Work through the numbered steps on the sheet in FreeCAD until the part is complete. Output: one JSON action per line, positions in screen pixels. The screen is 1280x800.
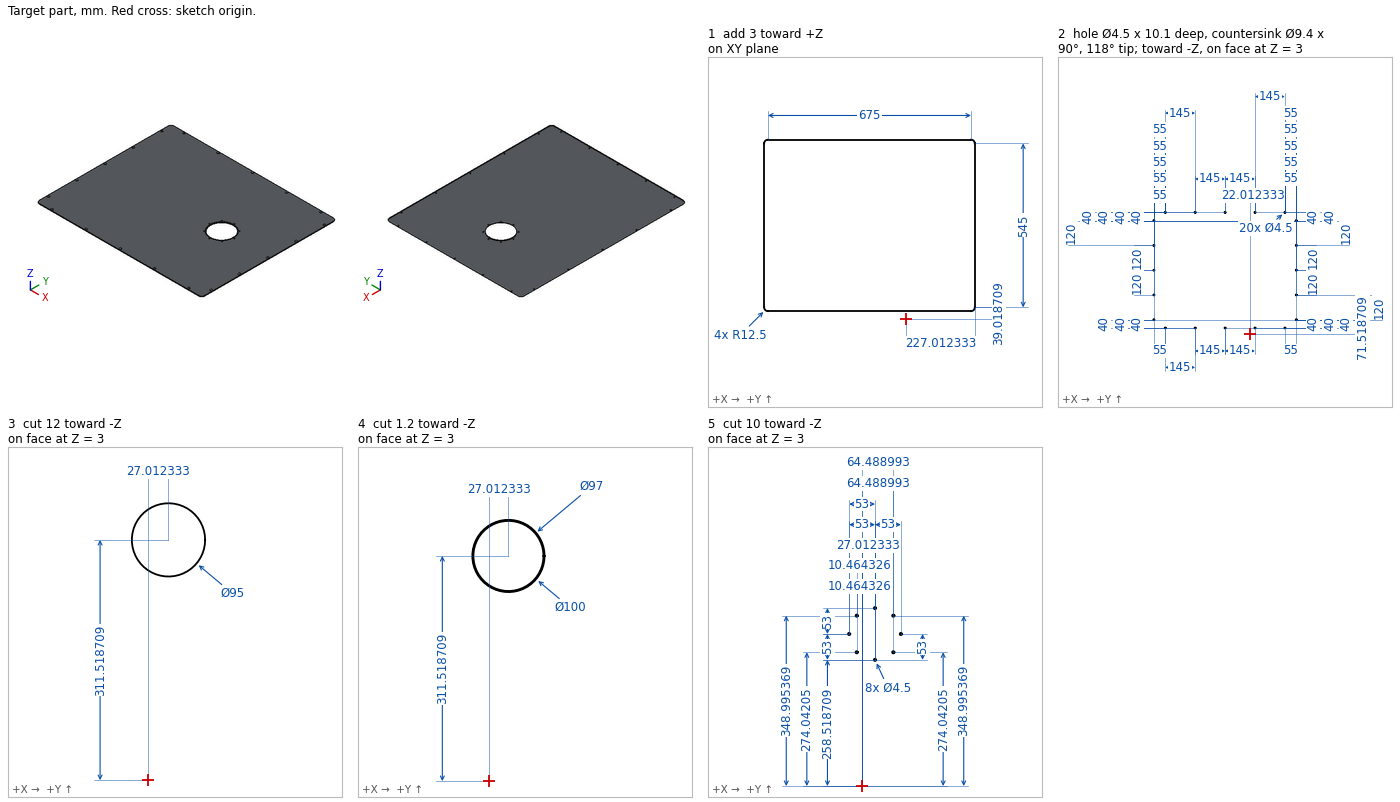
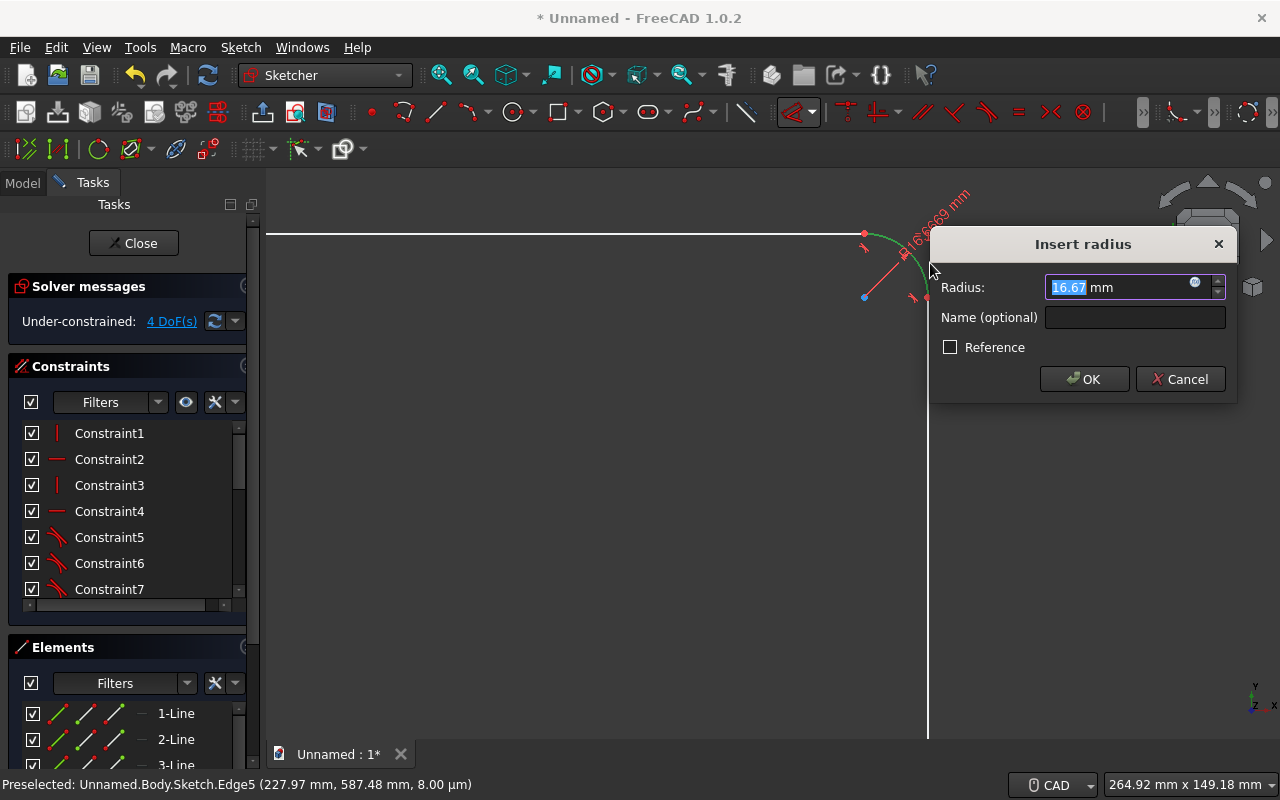
{"action": "type", "text": "12.5"}
{"action": "key", "text": "Return"}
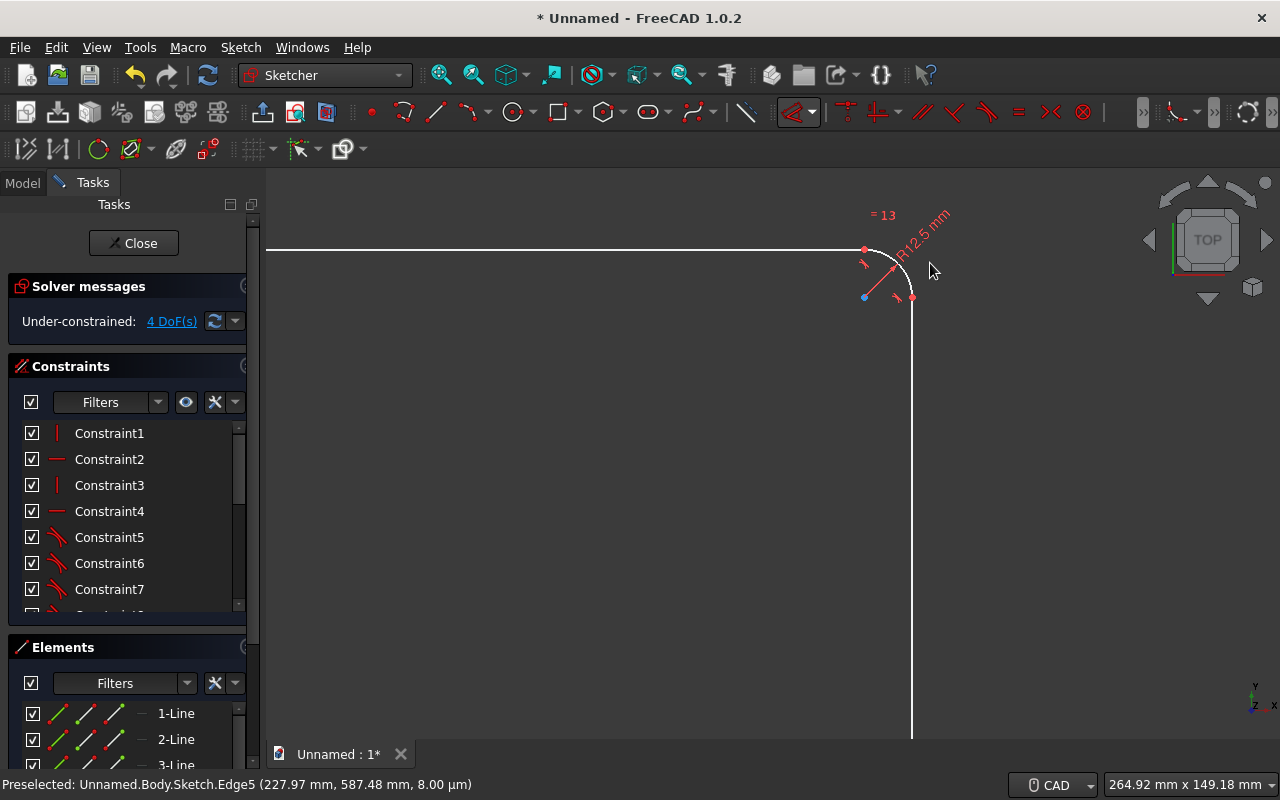
{"action": "scroll", "coordinate": [927, 270], "scroll_direction": "down", "scroll_amount": 9}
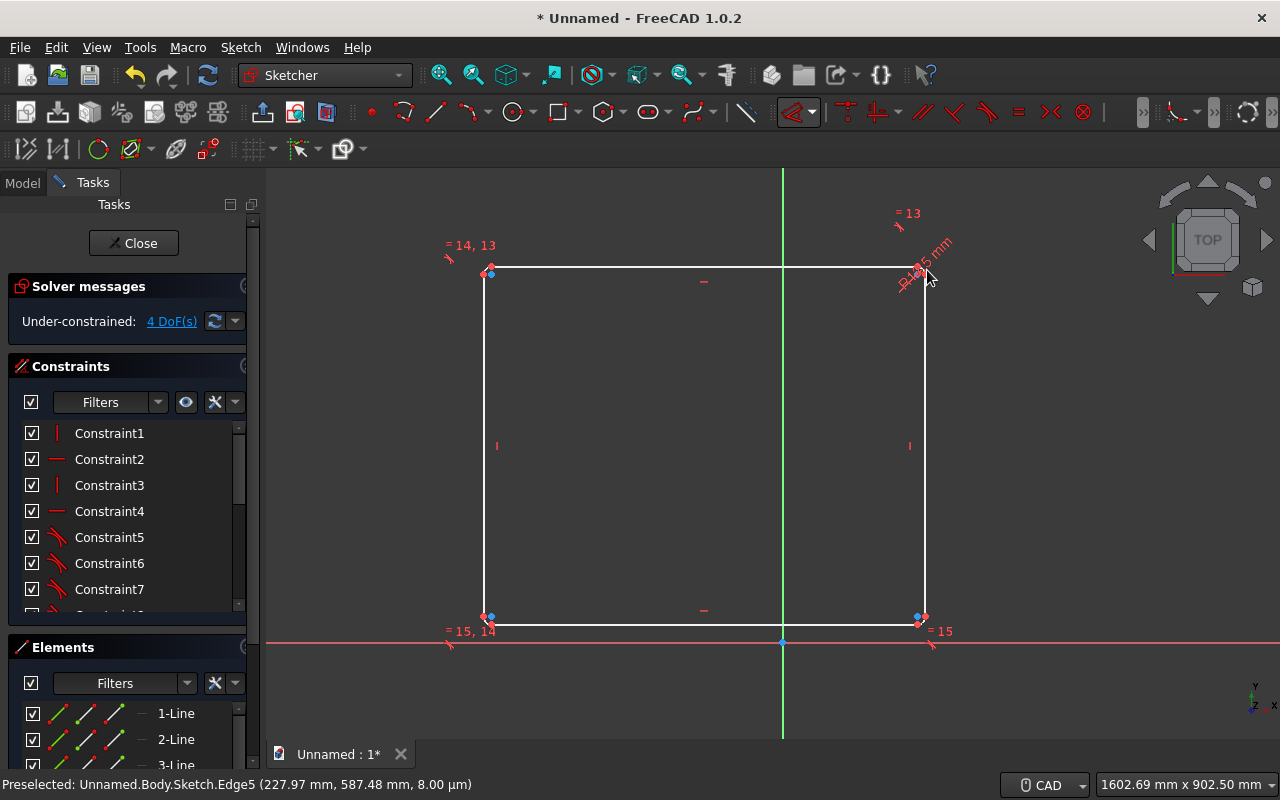
{"action": "left_click", "coordinate": [925, 514]}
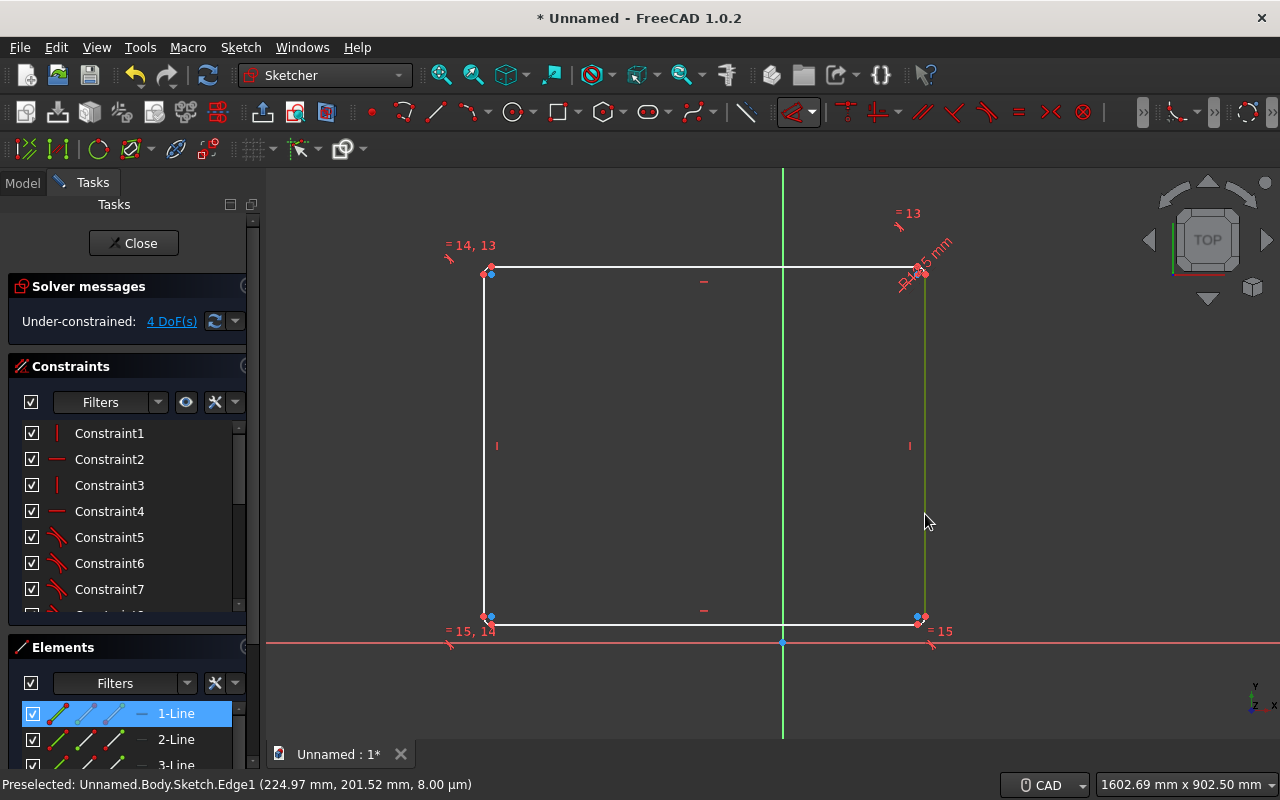
{"action": "key", "text": "i"}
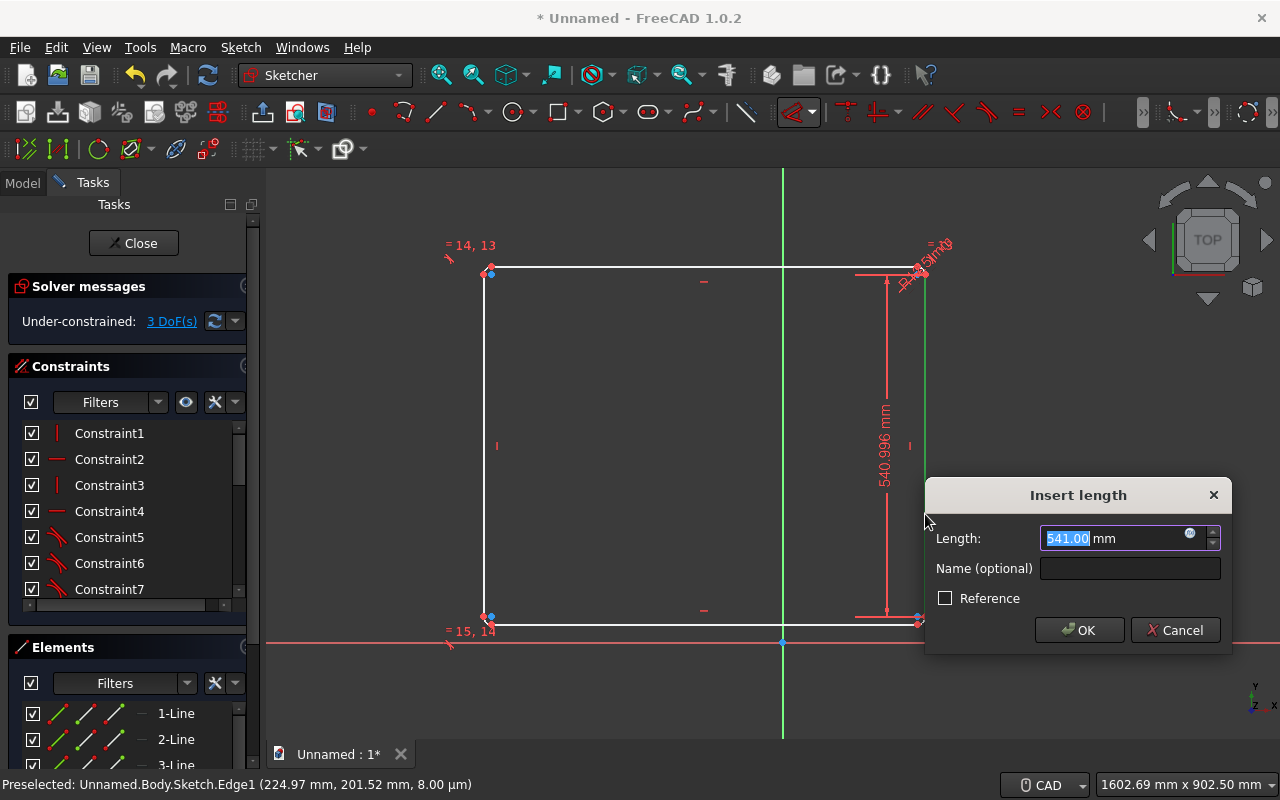
{"action": "type", "text": "545"}
{"action": "key", "text": "Return"}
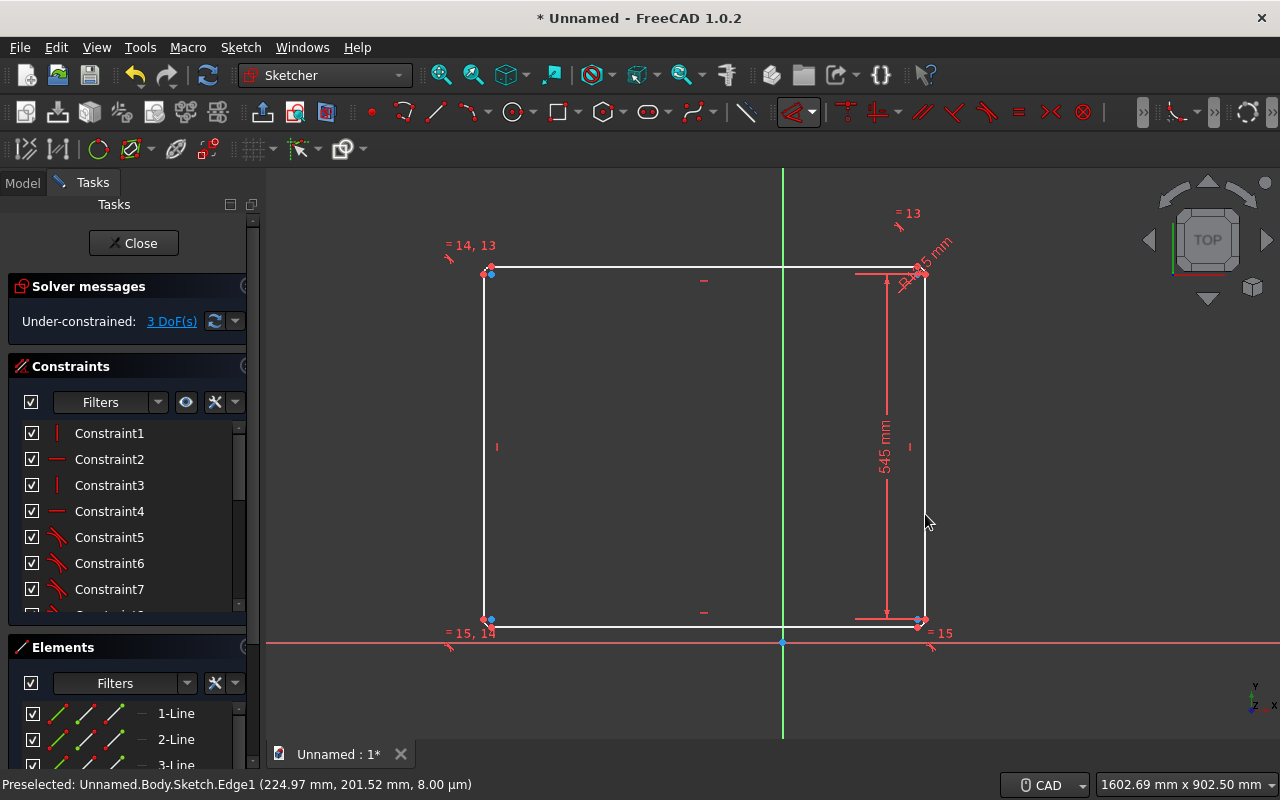
{"action": "left_click", "coordinate": [619, 267]}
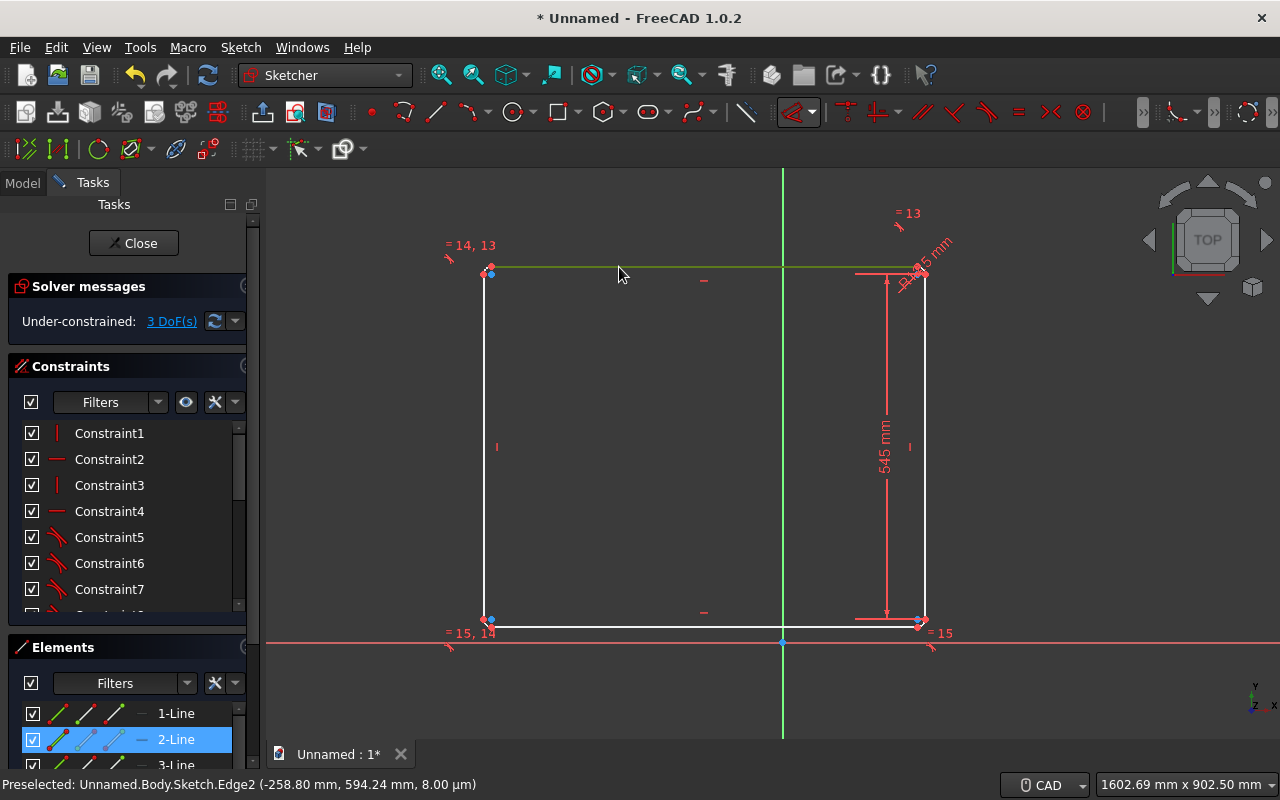
{"action": "left_click", "coordinate": [814, 112]}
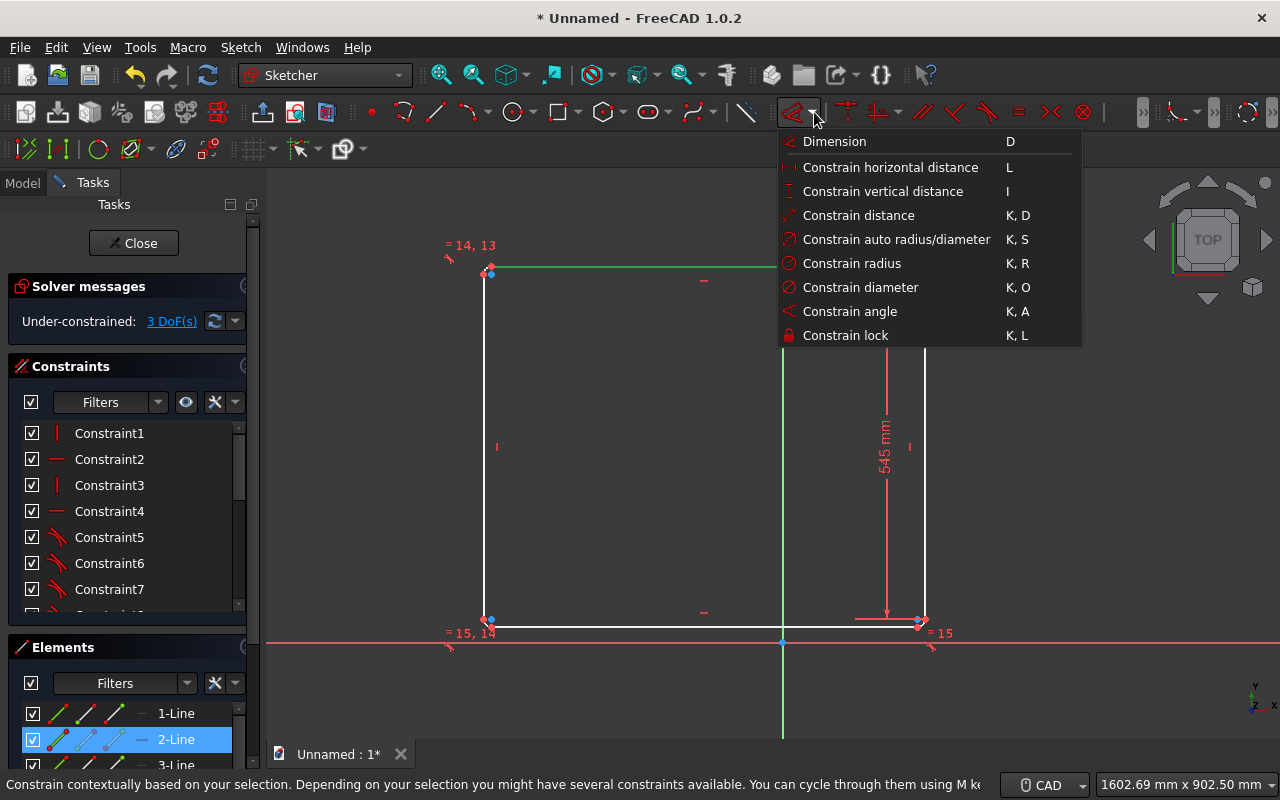
{"action": "left_click", "coordinate": [930, 167]}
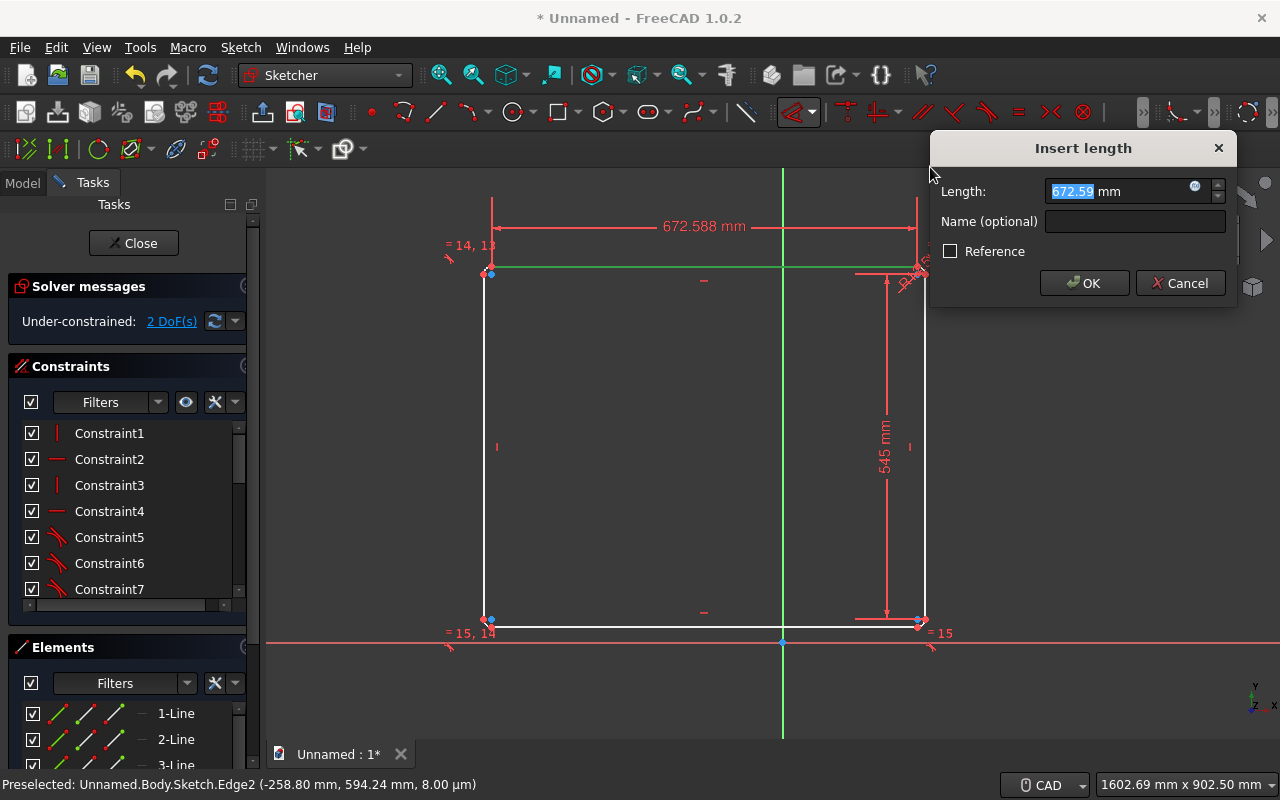
{"action": "type", "text": "675"}
{"action": "key", "text": "Return"}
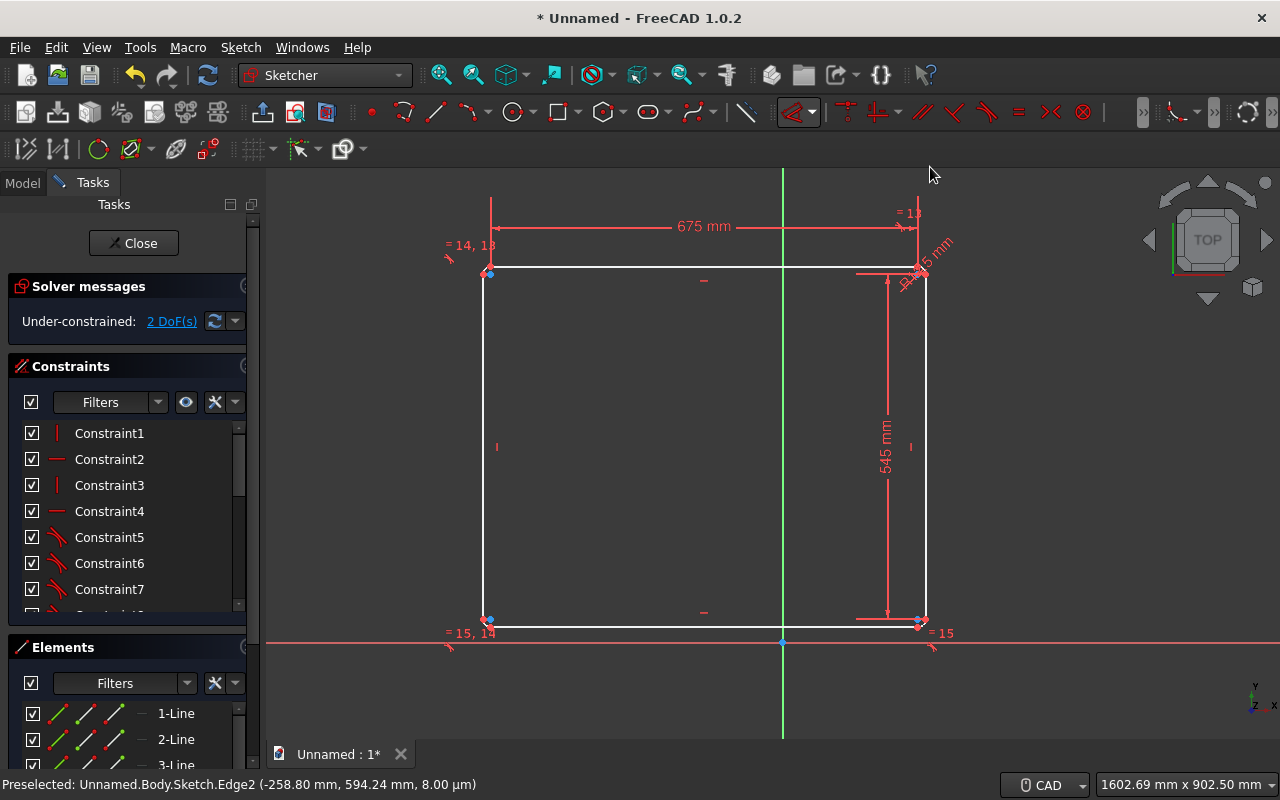
{"action": "scroll", "coordinate": [926, 619], "scroll_direction": "up", "scroll_amount": 3}